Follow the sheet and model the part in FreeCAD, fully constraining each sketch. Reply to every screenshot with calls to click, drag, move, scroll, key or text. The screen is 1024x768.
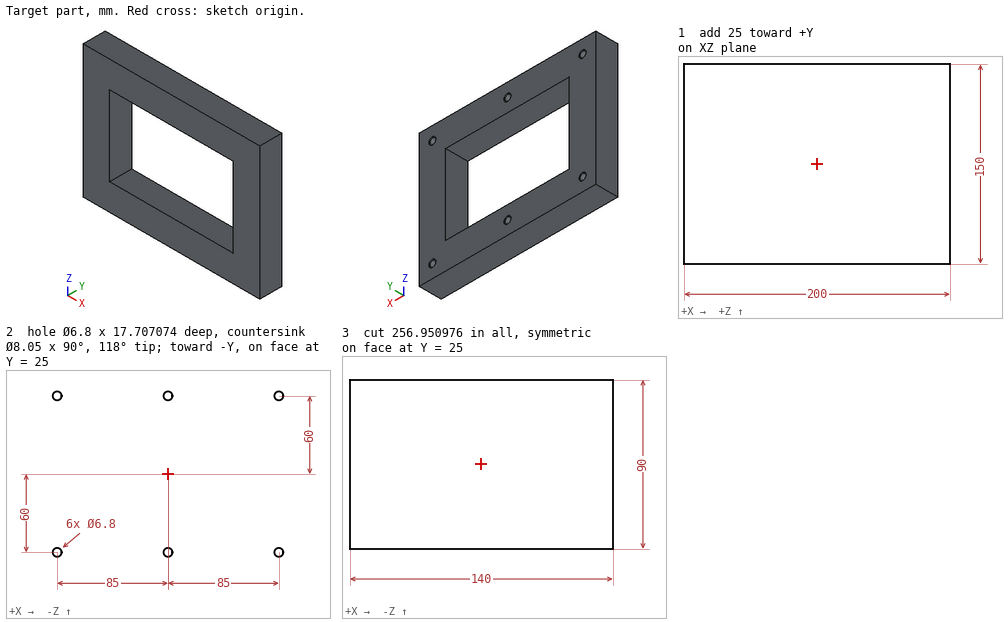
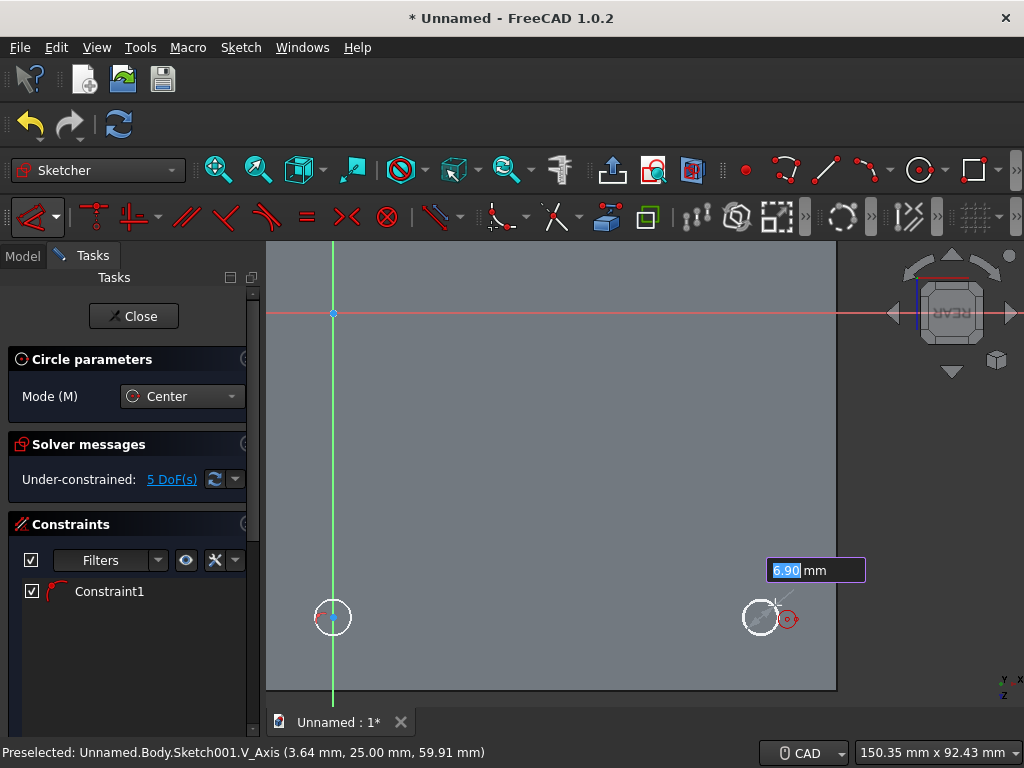
click(774, 603)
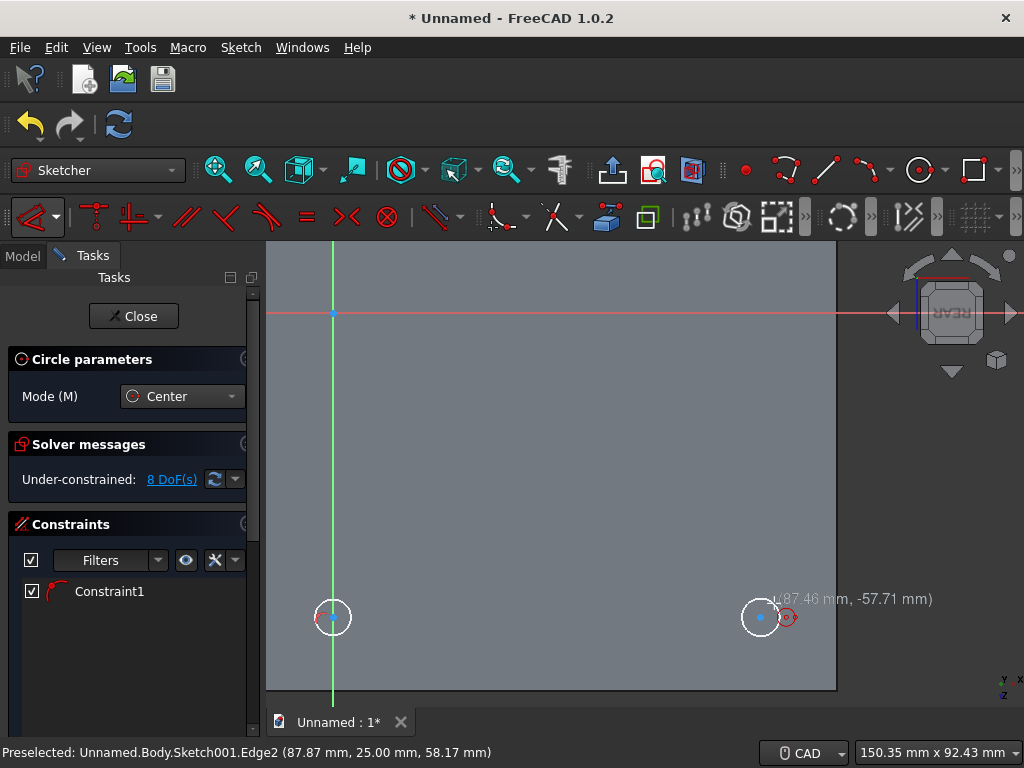
scroll(775, 605, down, 4)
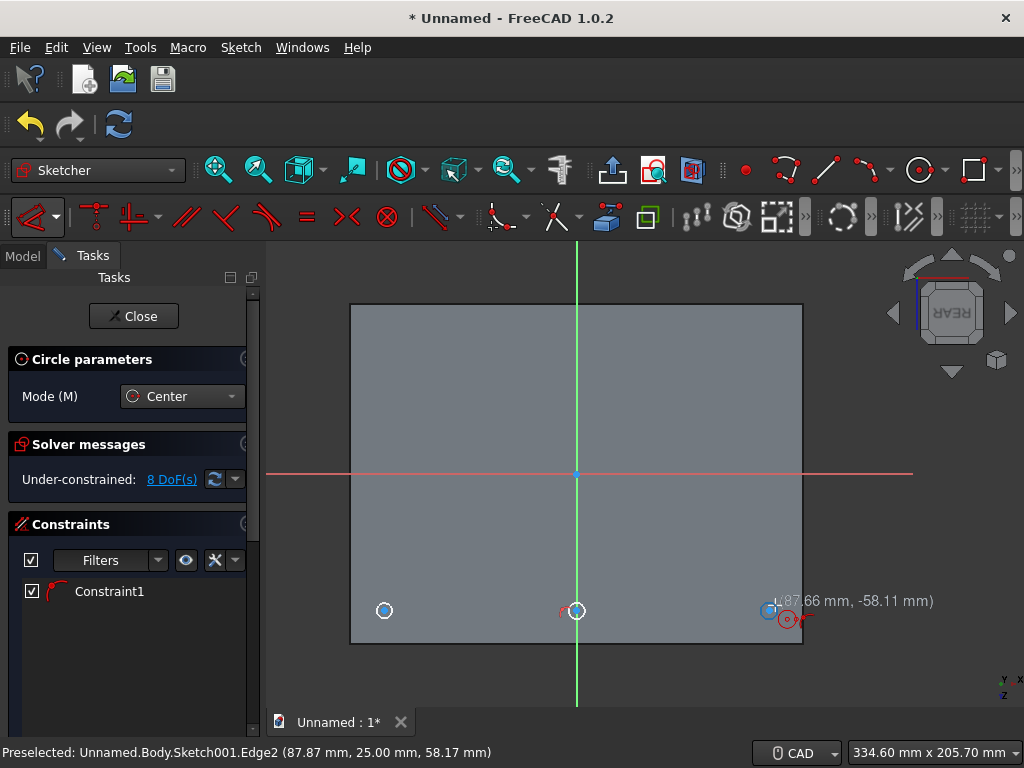
scroll(769, 338, up, 6)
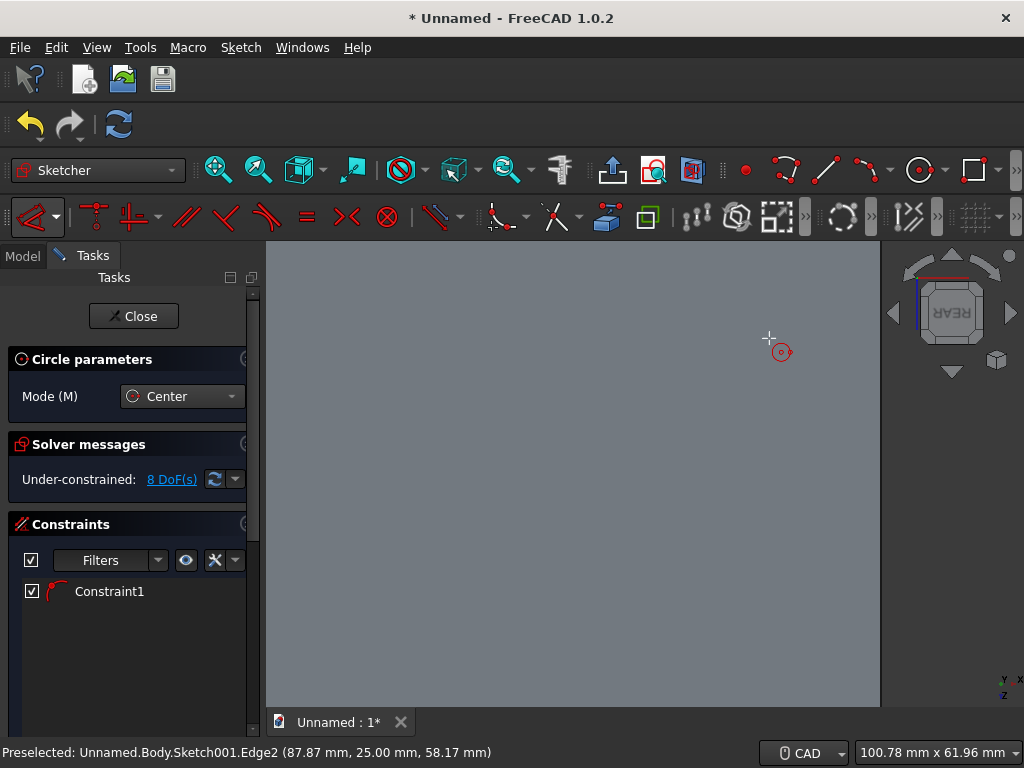
scroll(769, 338, down, 6)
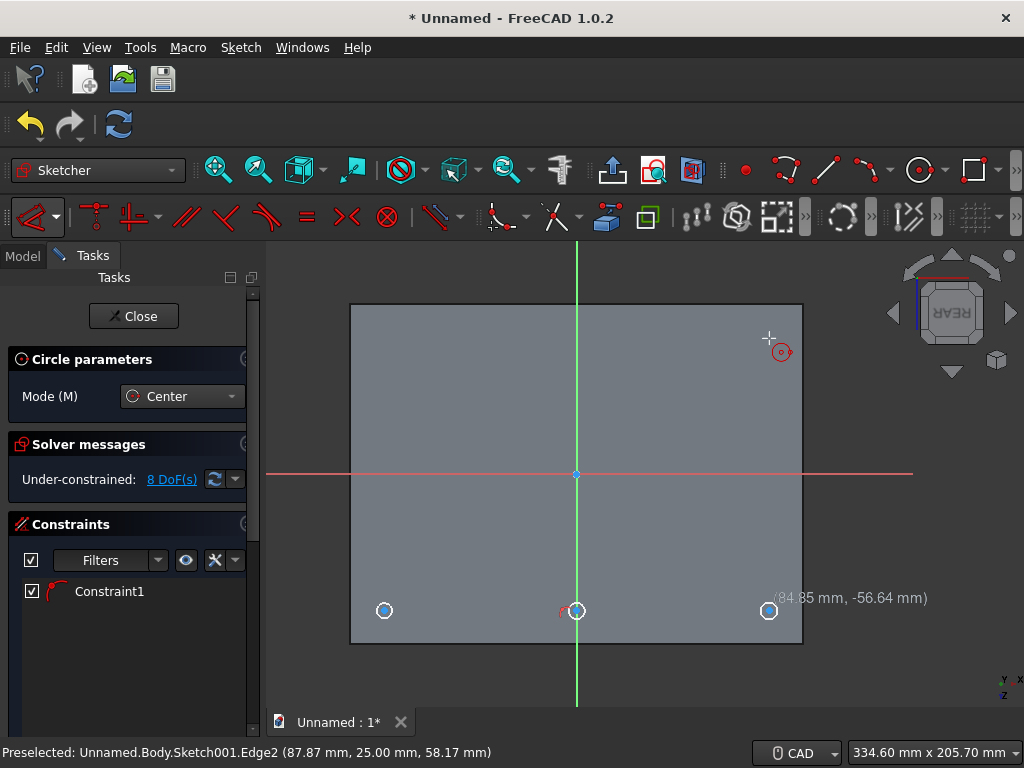
click(769, 338)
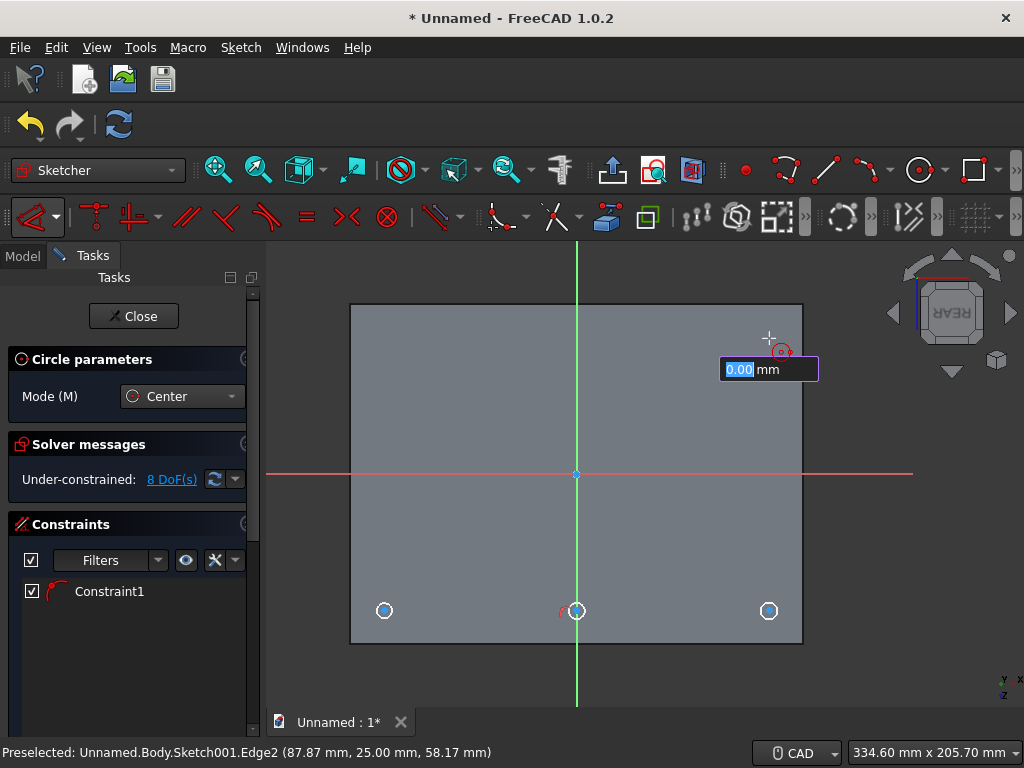
scroll(775, 333, up, 4)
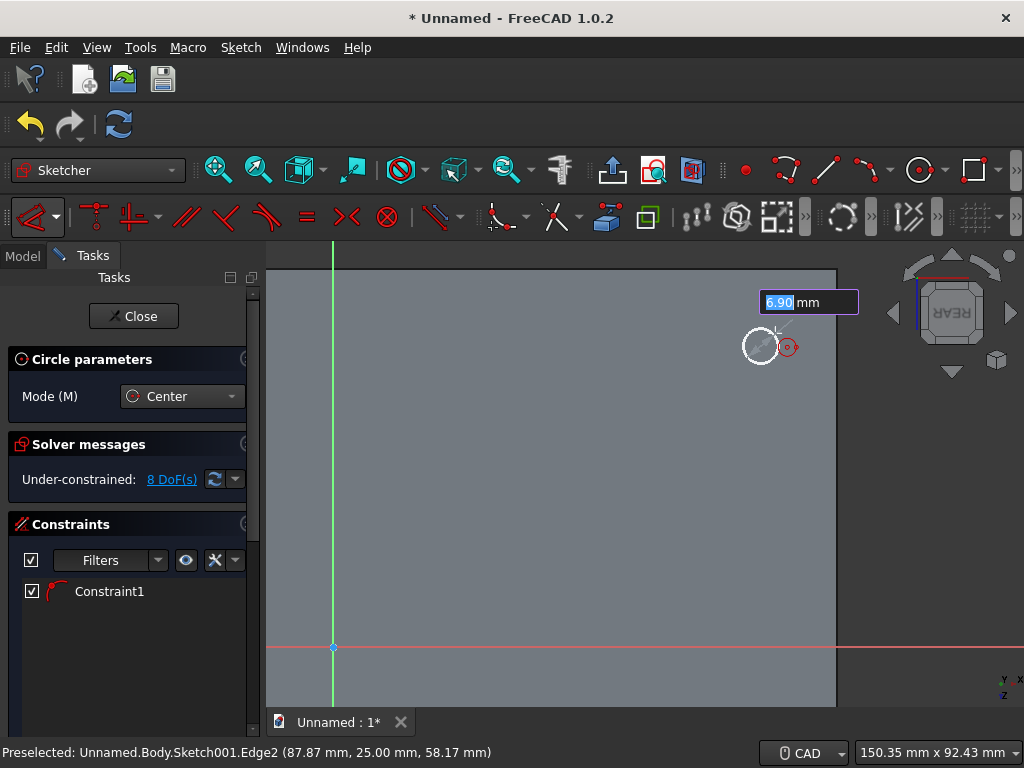
click(774, 332)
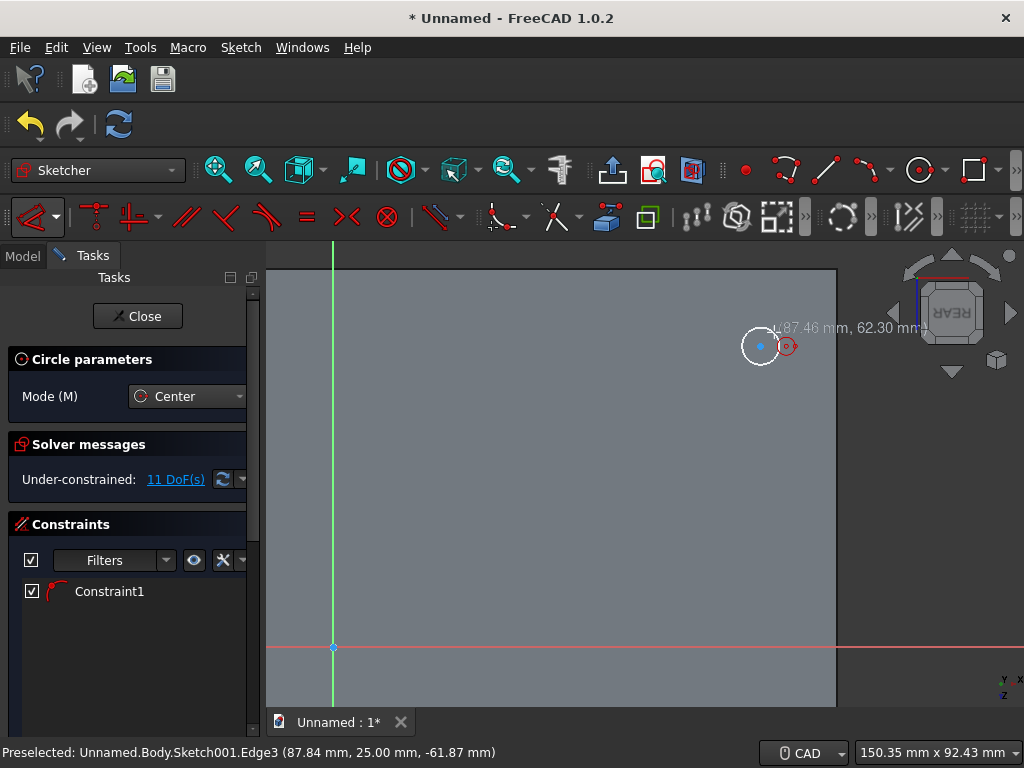
scroll(333, 345, up, 2)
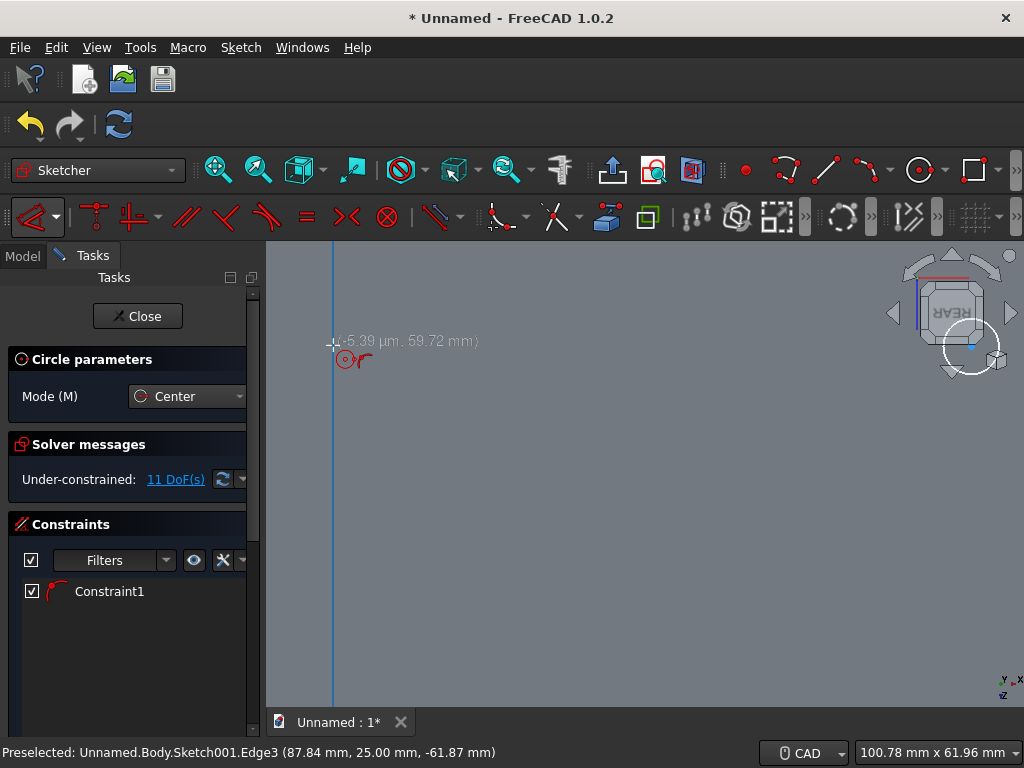
scroll(681, 335, down, 6)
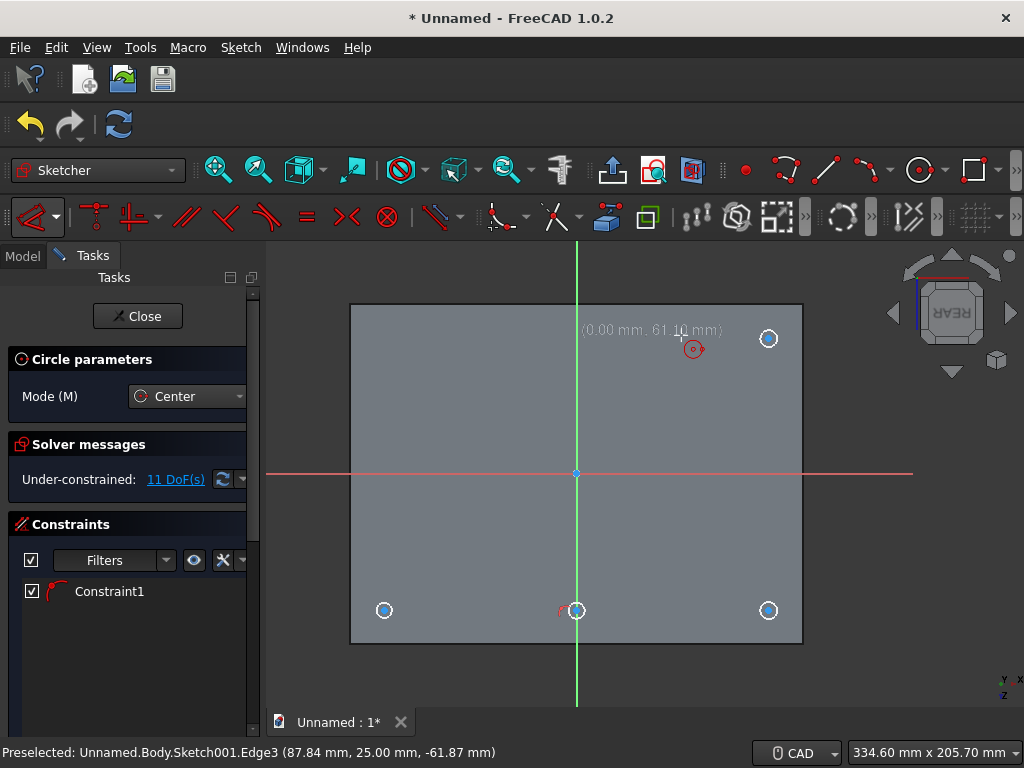
click(577, 338)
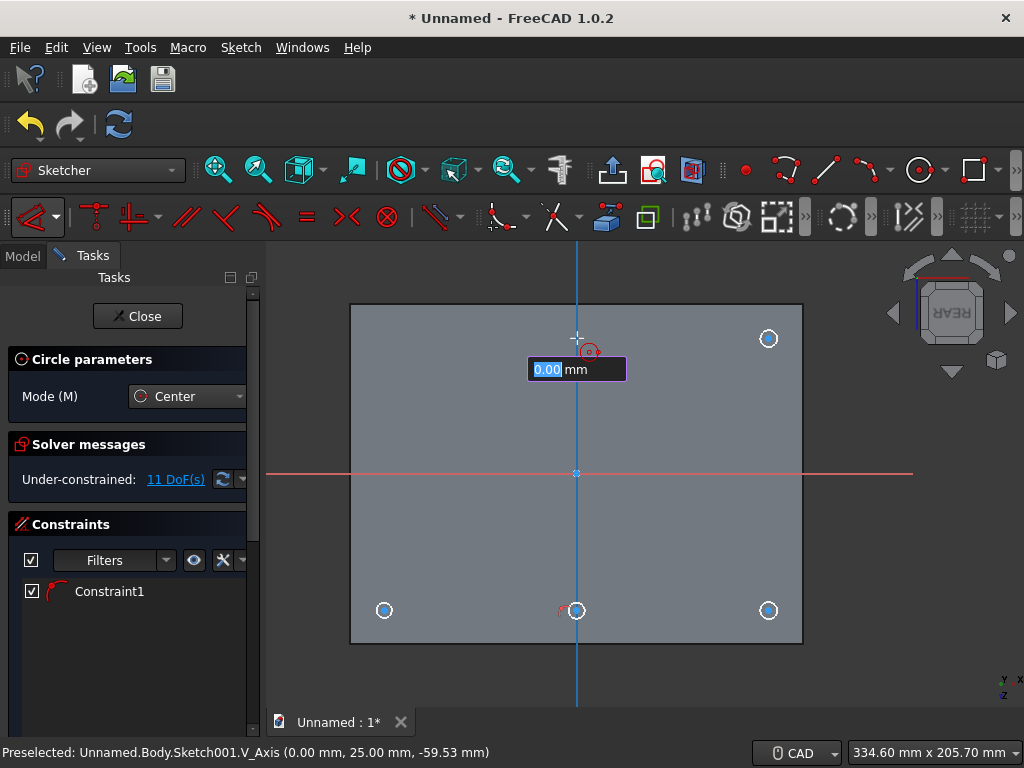
scroll(584, 335, up, 4)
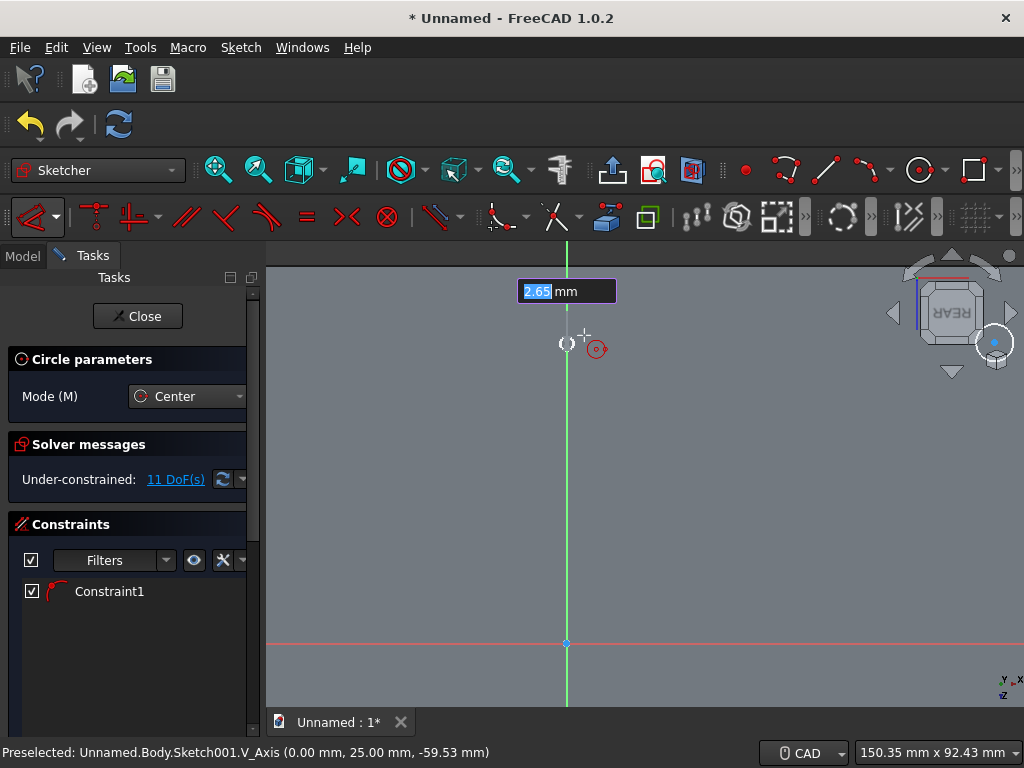
click(583, 335)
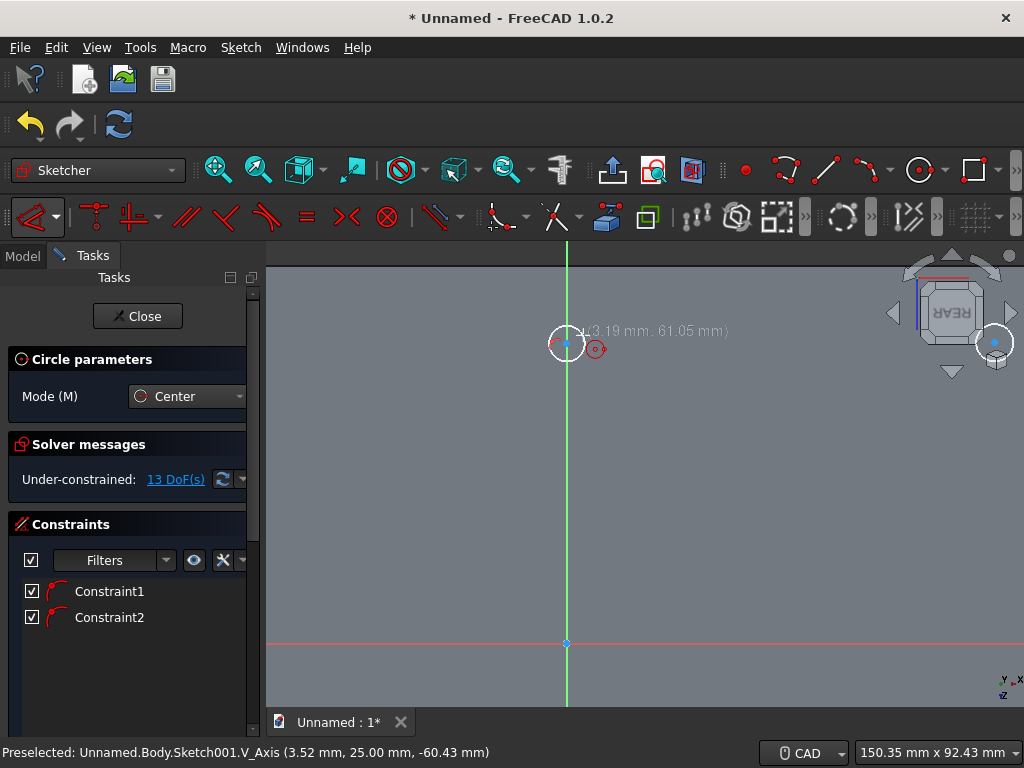
scroll(584, 335, down, 4)